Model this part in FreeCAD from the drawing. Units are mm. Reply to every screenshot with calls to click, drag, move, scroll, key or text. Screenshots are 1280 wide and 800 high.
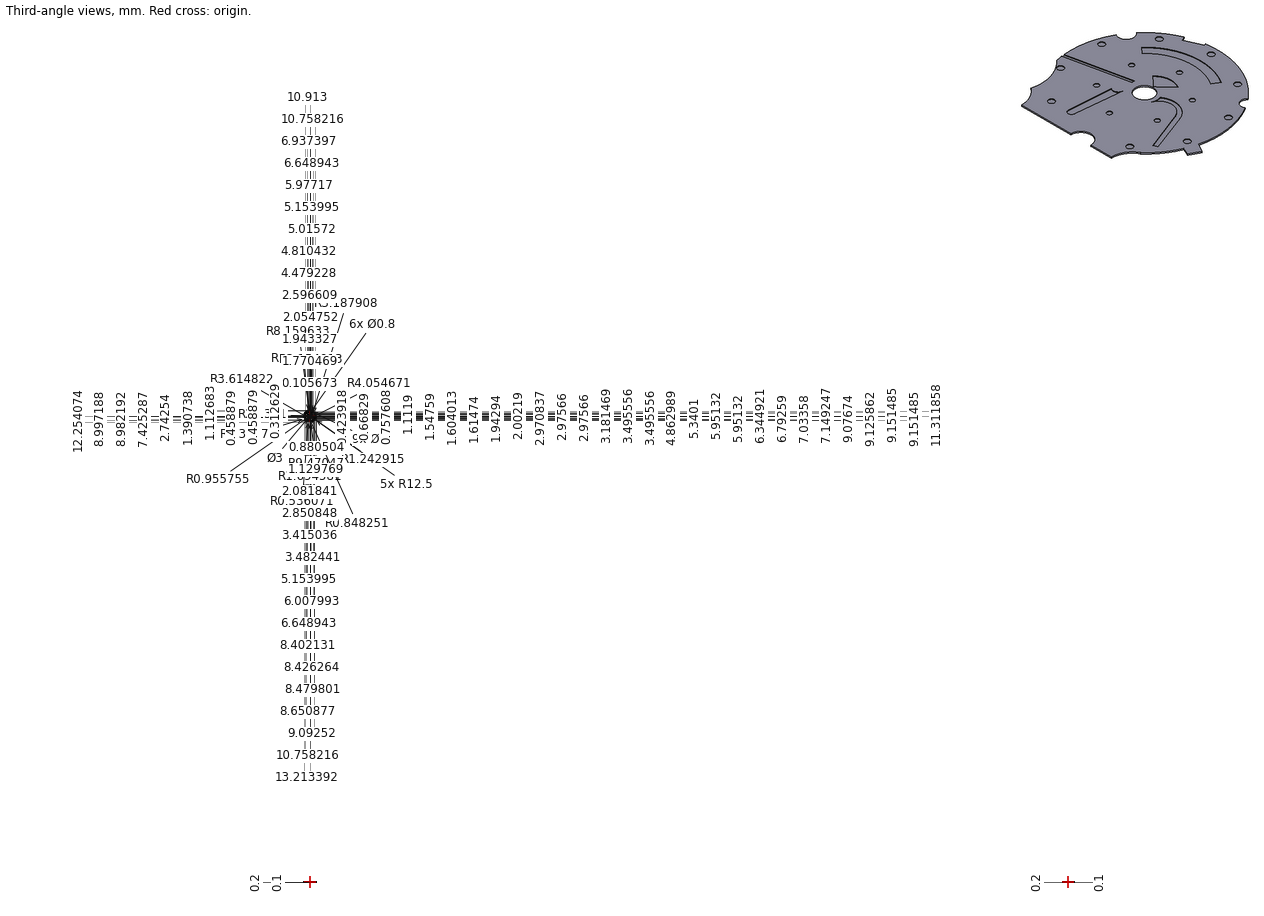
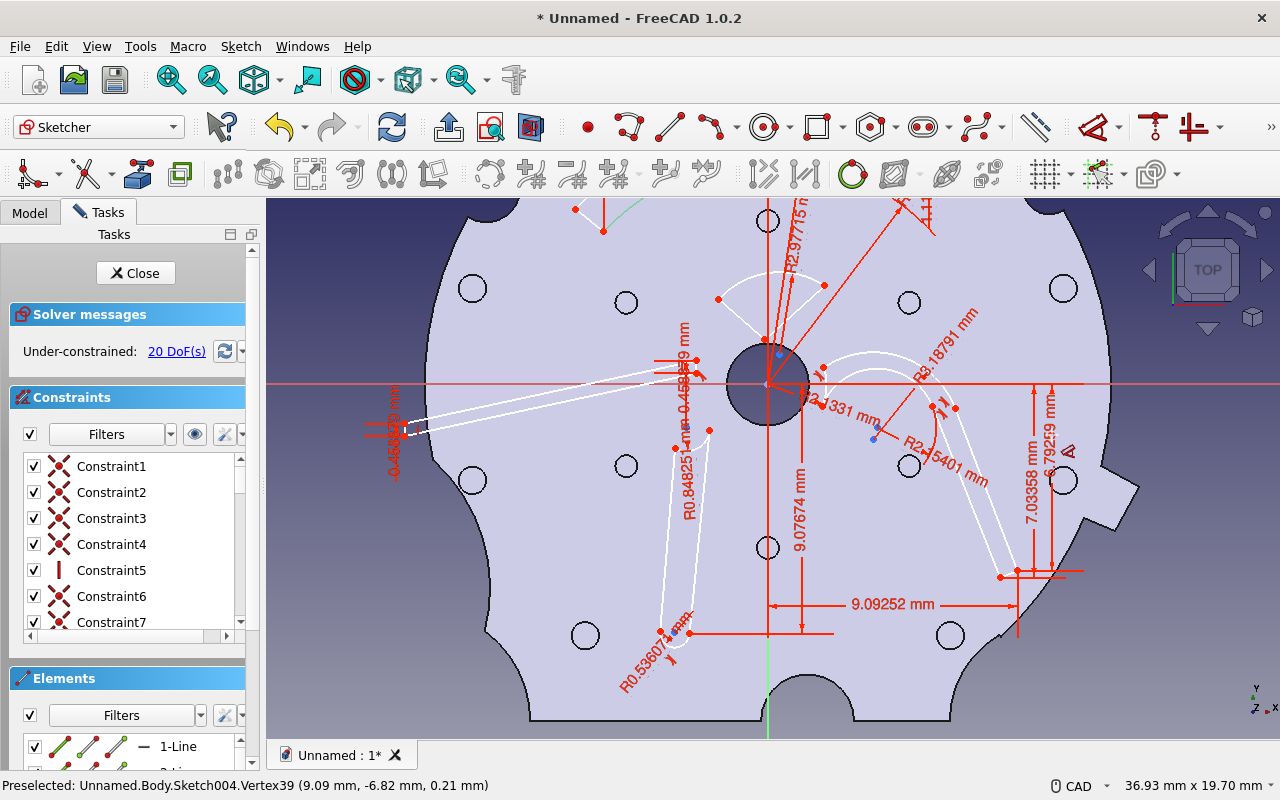
scroll(824, 368, up, 4)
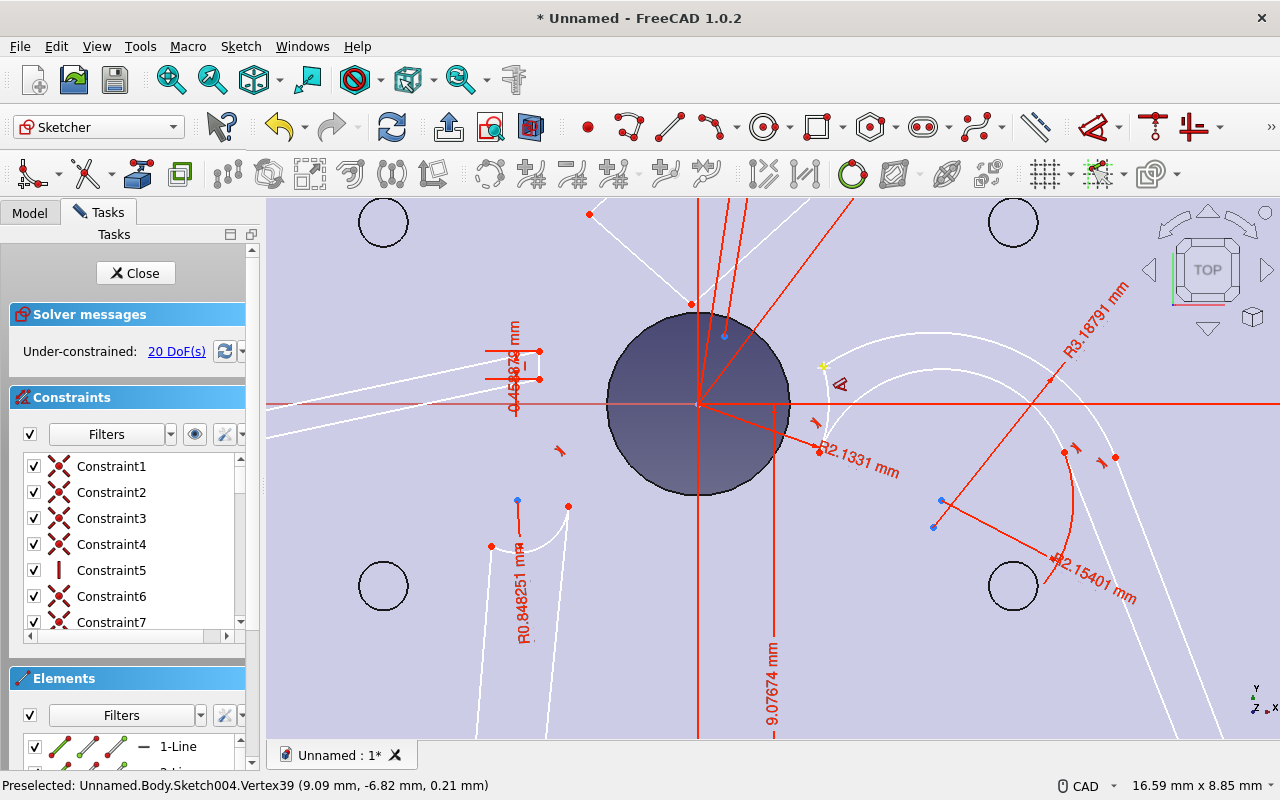
click(823, 367)
click(857, 377)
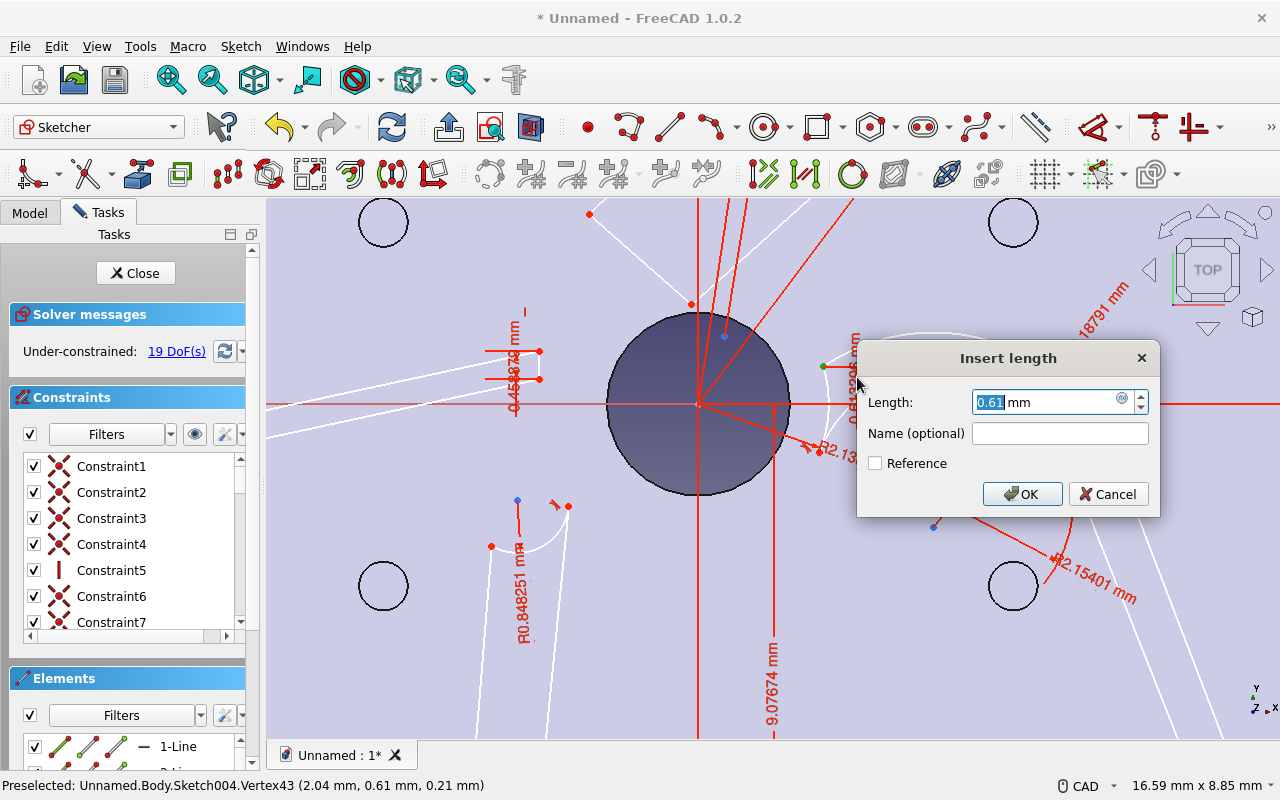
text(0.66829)
key(Return)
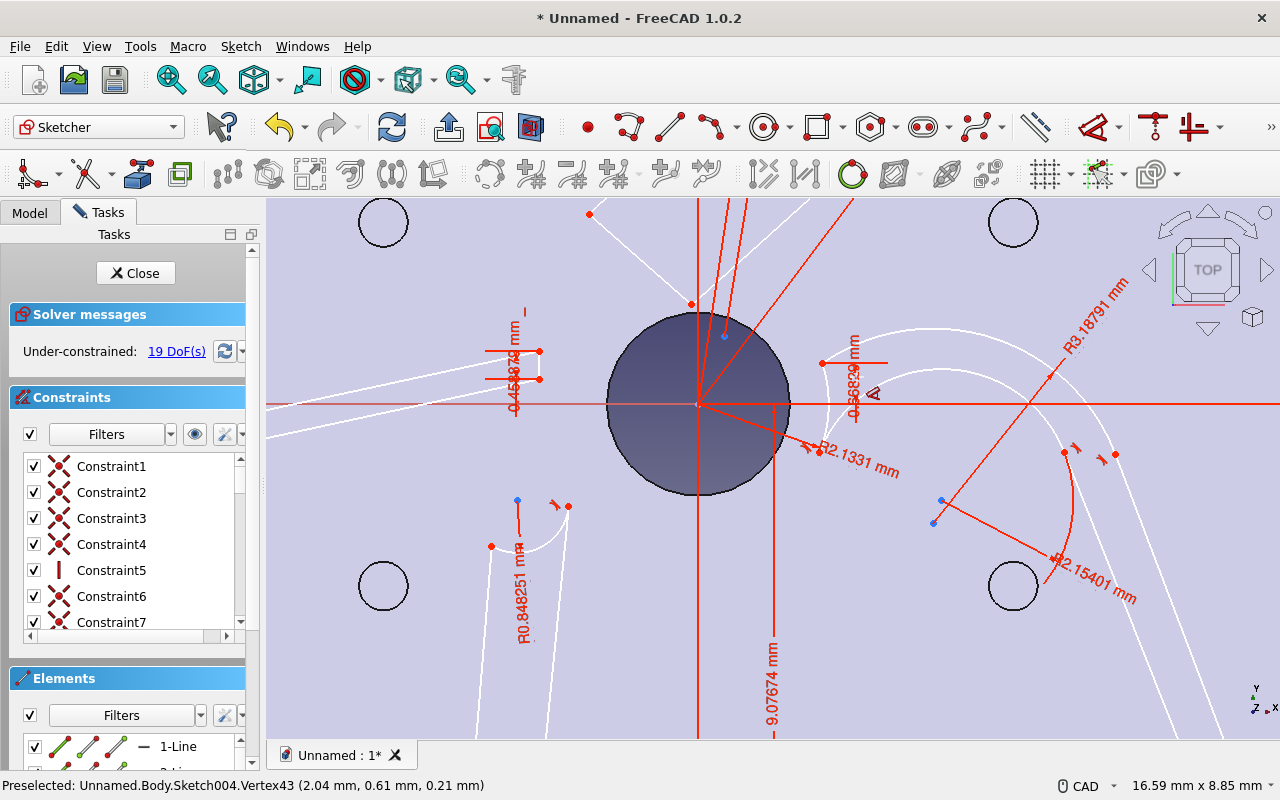
click(620, 242)
click(726, 247)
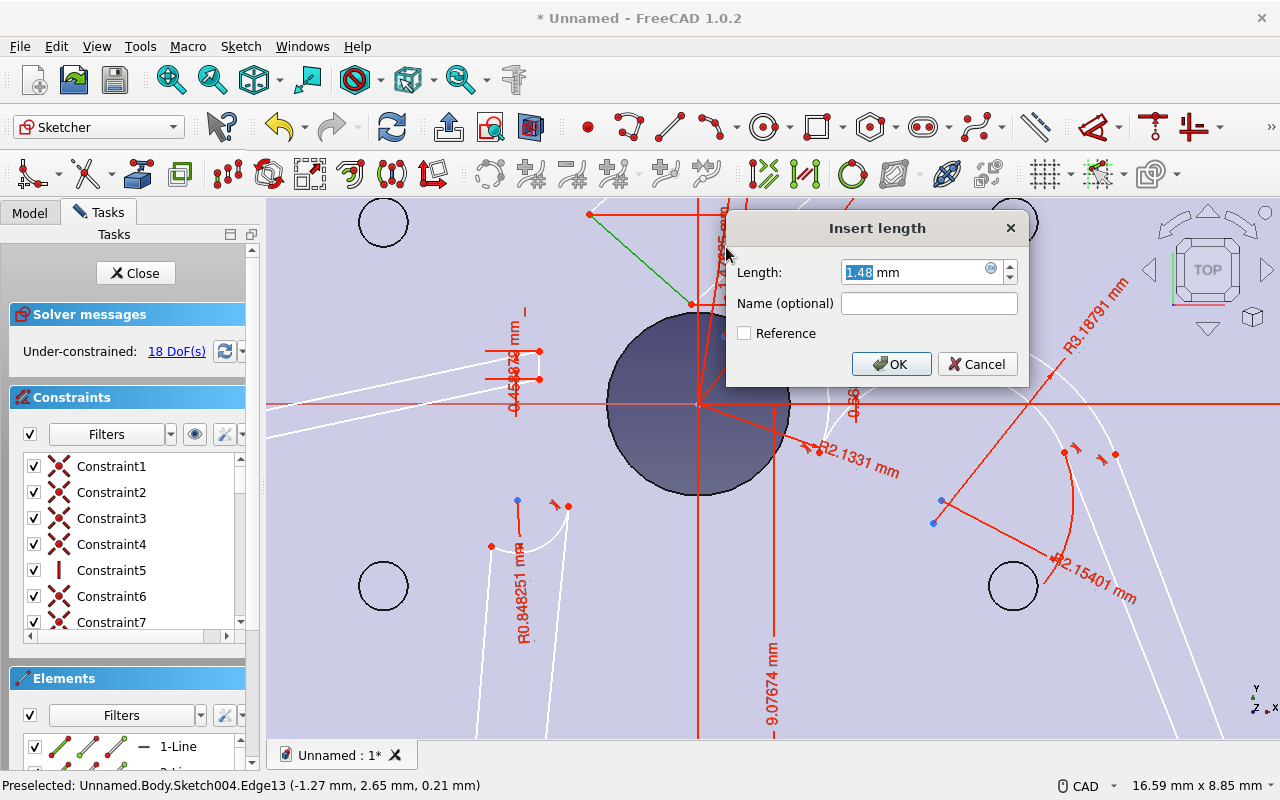
text(1.54759)
key(Return)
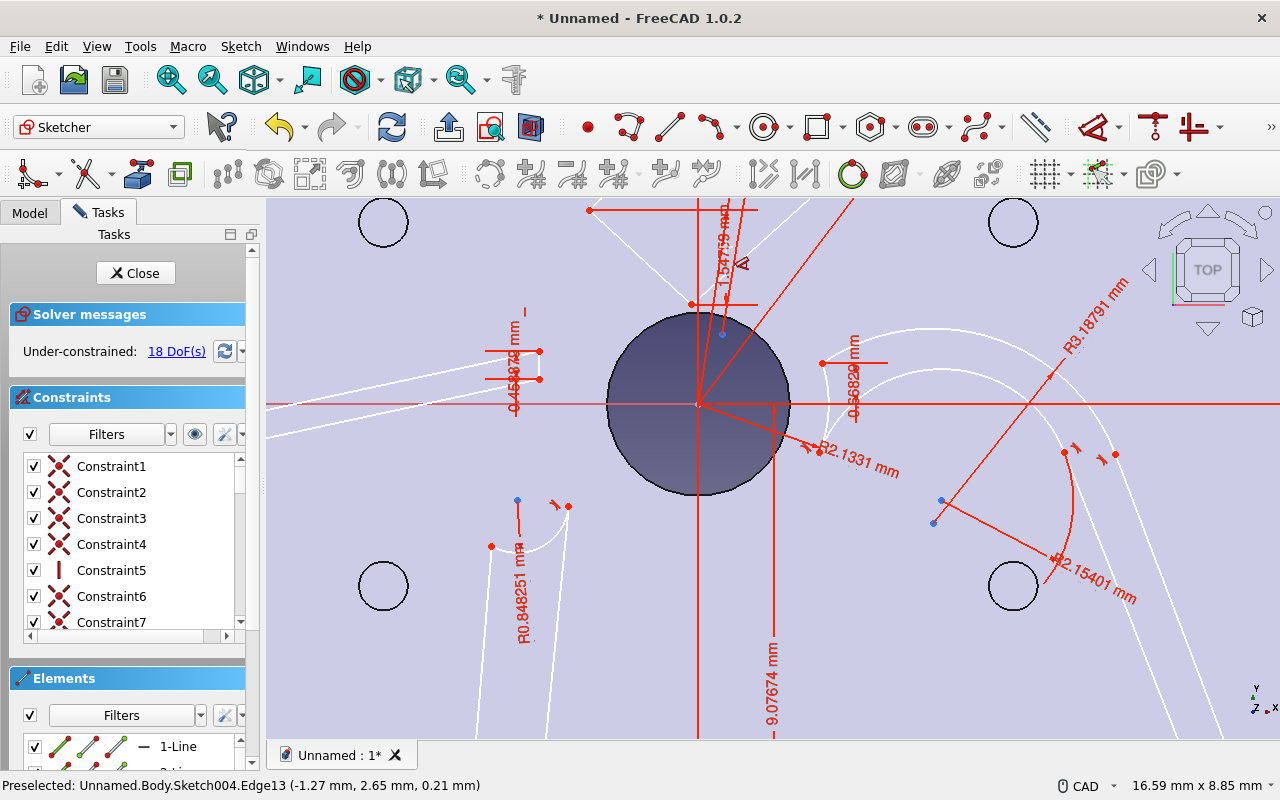
click(732, 269)
click(859, 265)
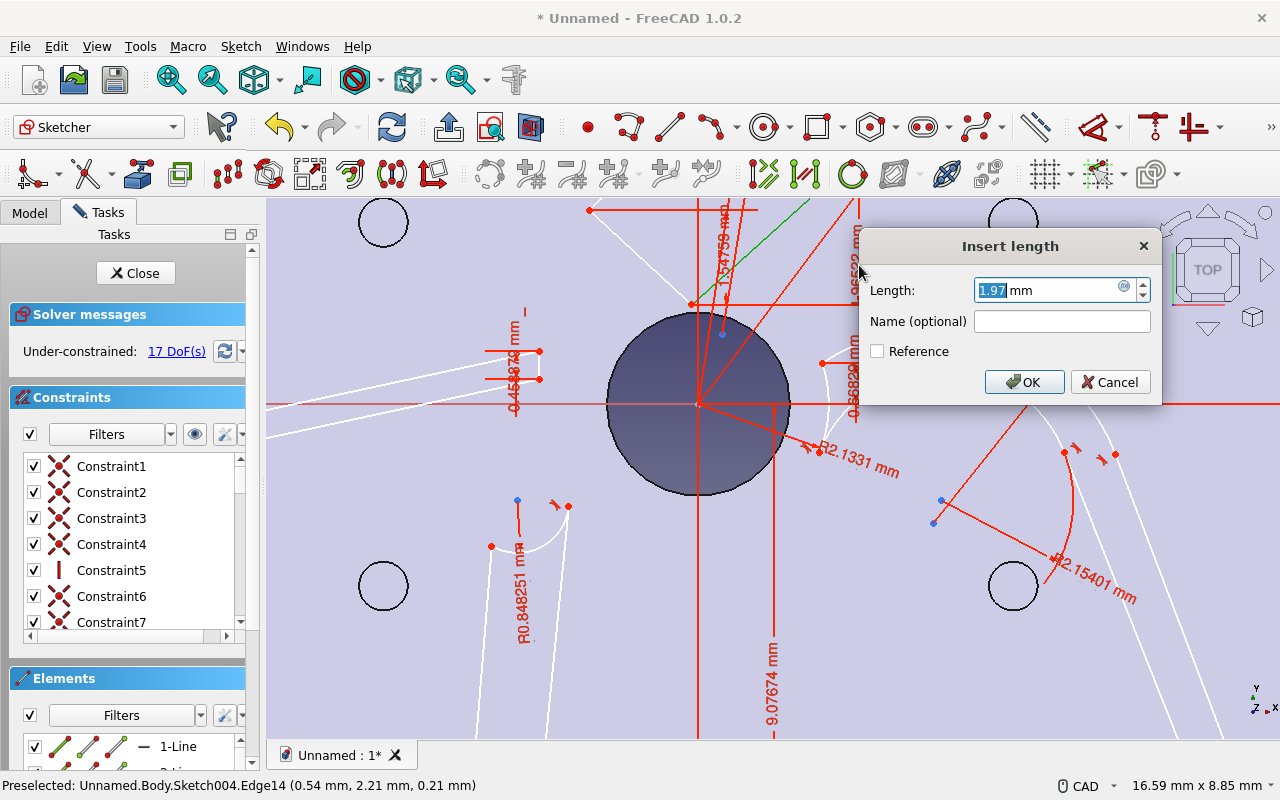
text(2.00219)
key(Return)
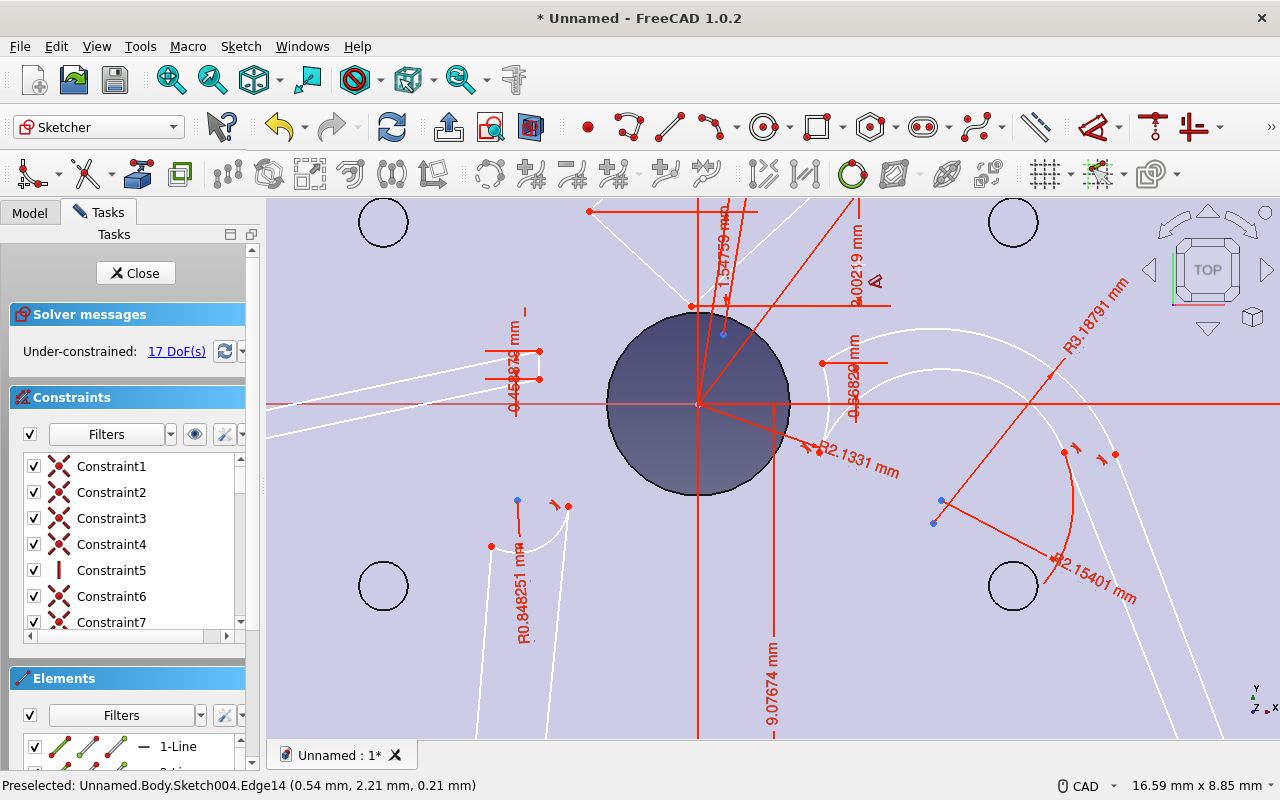
click(933, 523)
click(967, 464)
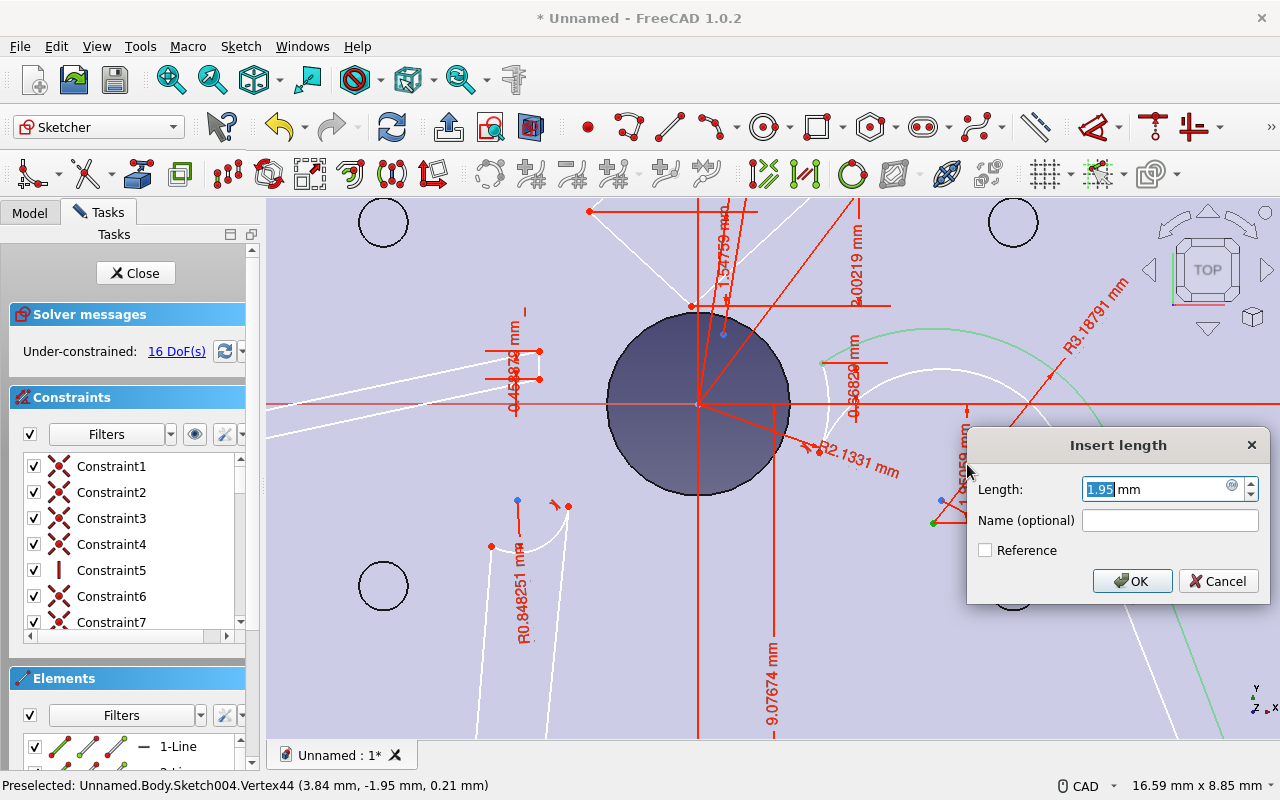
text(1.94294)
key(Return)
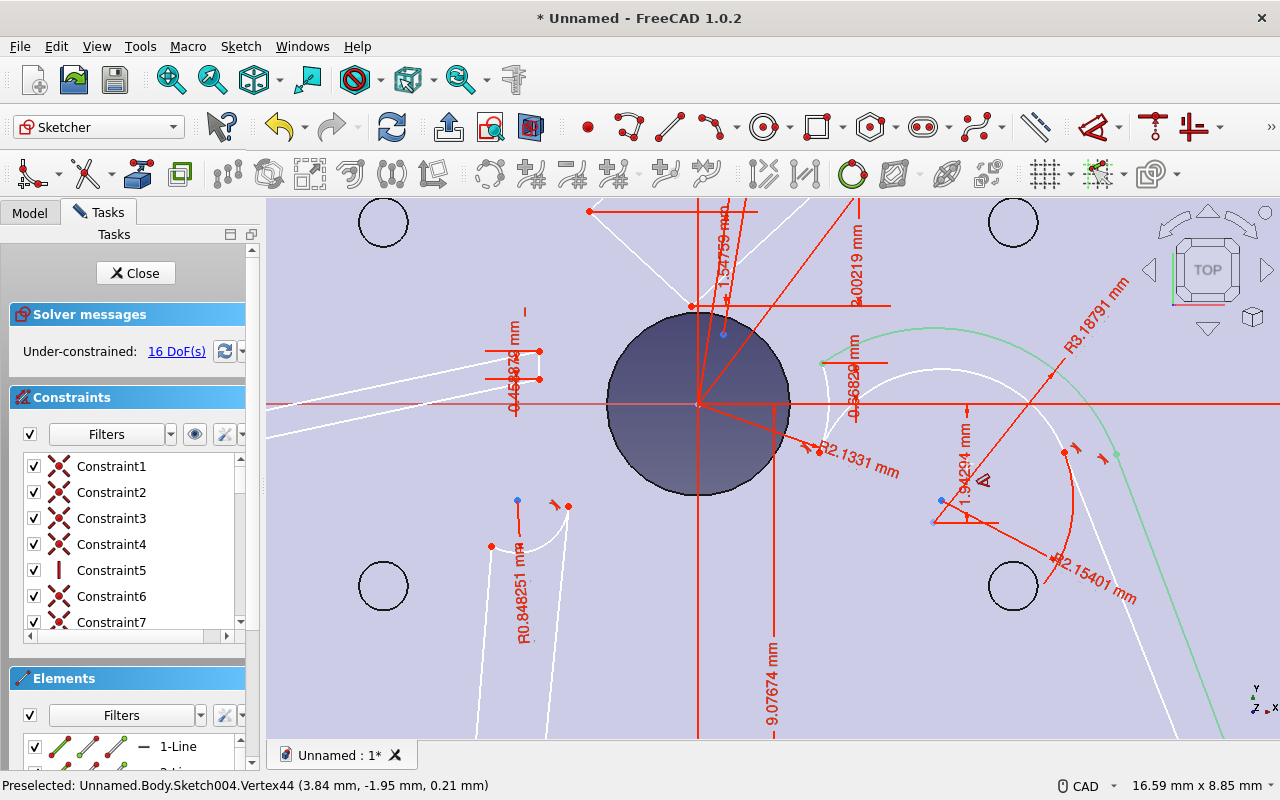
scroll(761, 494, down, 6)